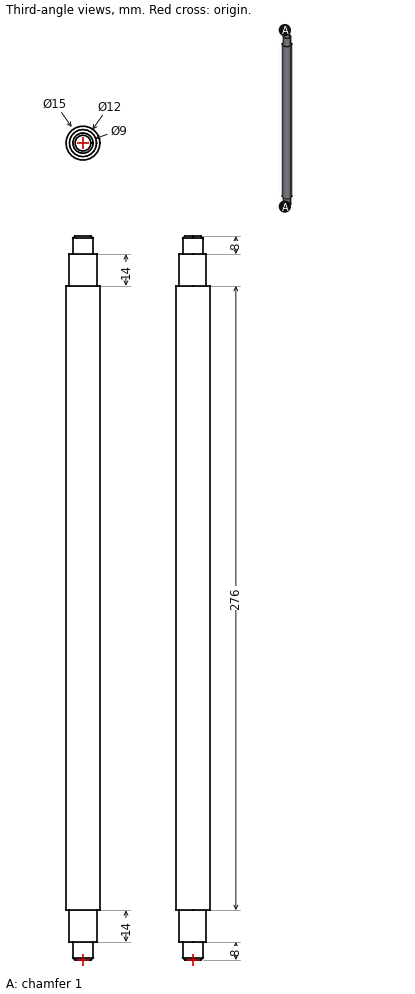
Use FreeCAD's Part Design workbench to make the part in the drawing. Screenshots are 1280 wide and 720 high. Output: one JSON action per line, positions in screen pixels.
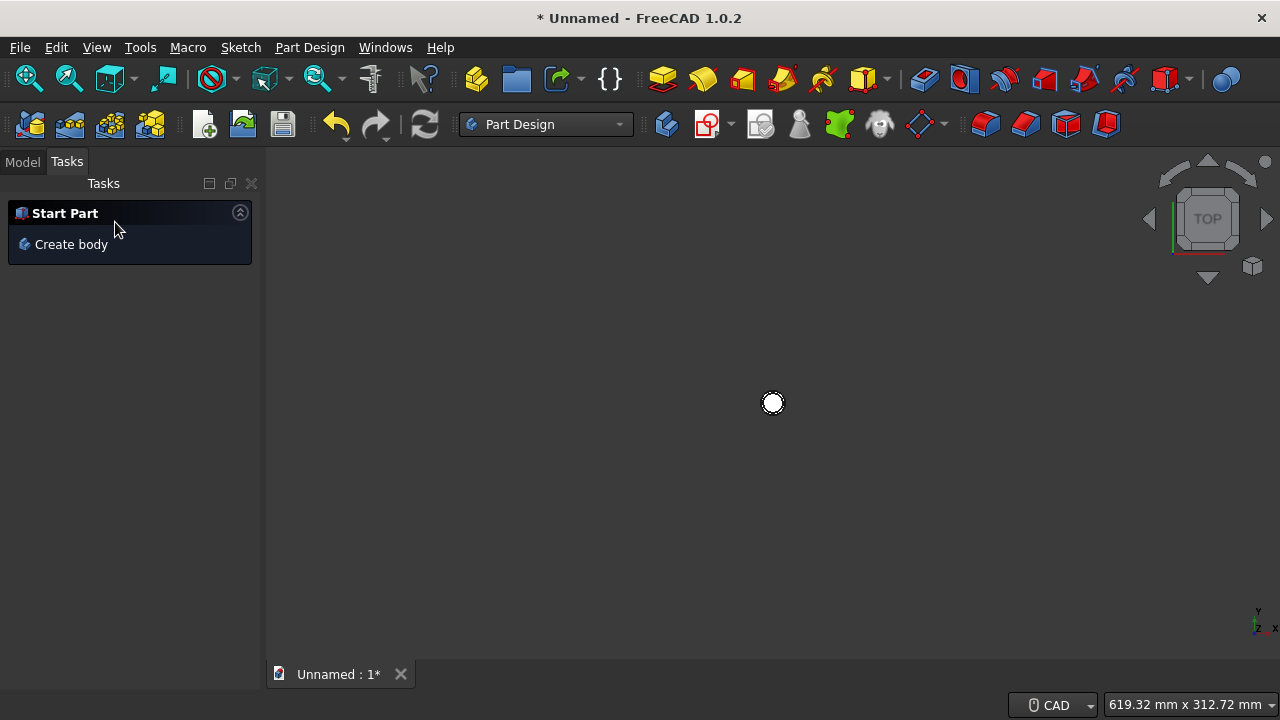
{"action": "left_click", "coordinate": [773, 402]}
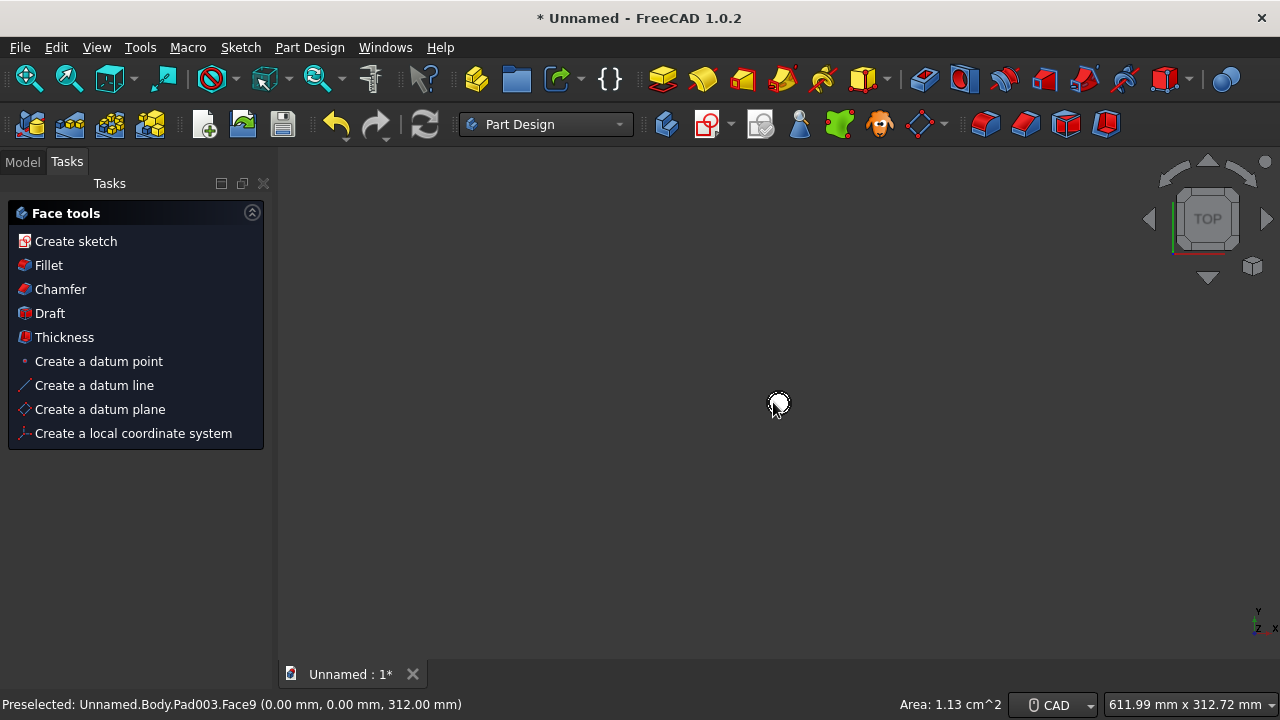
{"action": "left_click", "coordinate": [708, 124]}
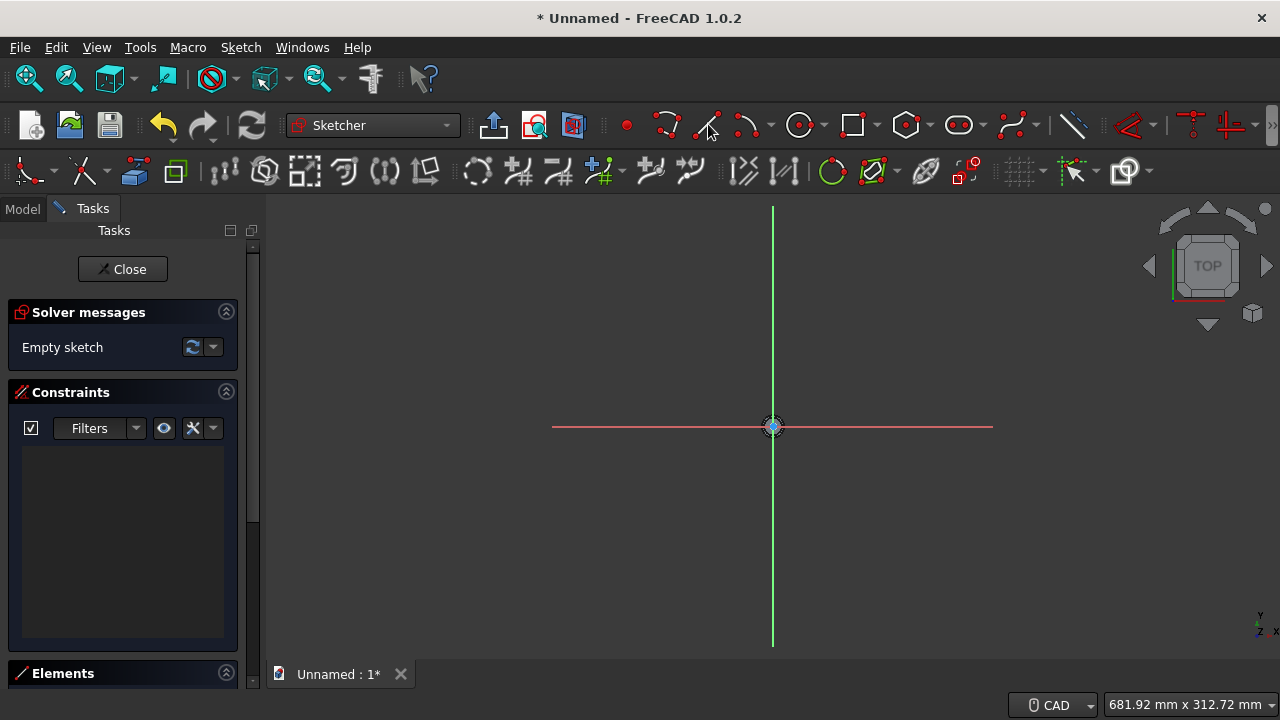
{"action": "scroll", "coordinate": [777, 426], "scroll_direction": "up", "scroll_amount": 15}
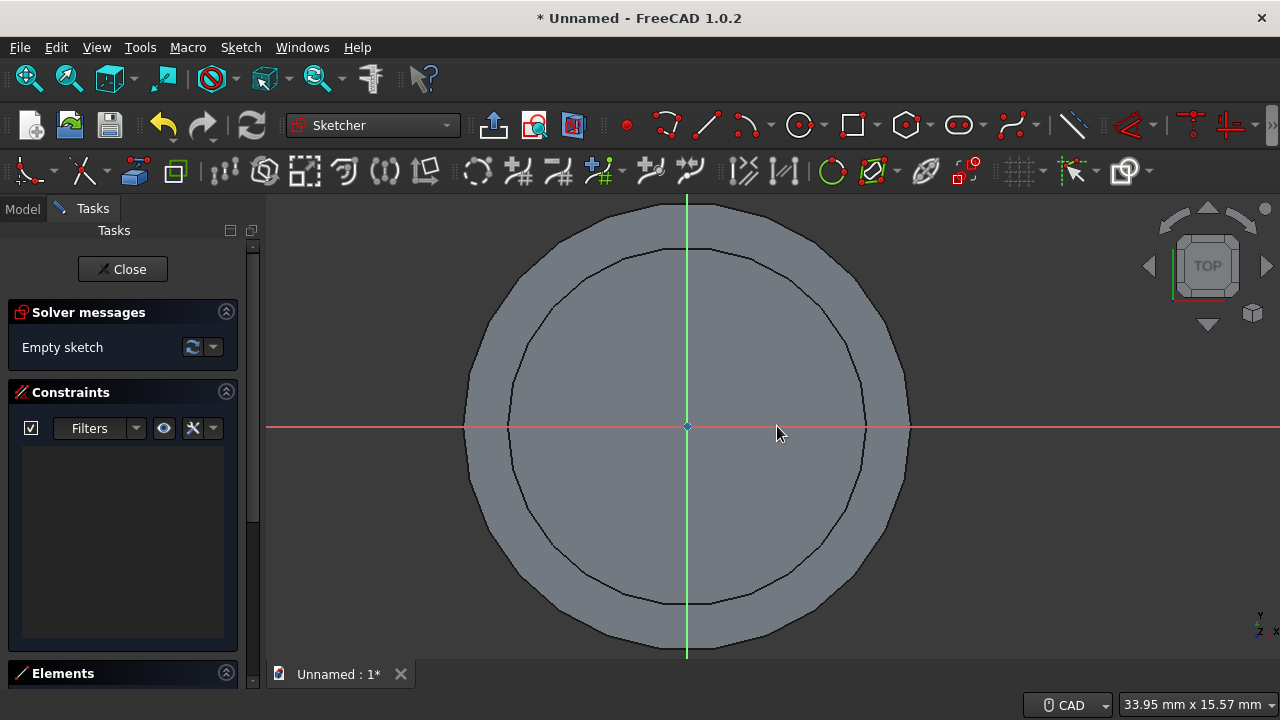
{"action": "left_click", "coordinate": [800, 126]}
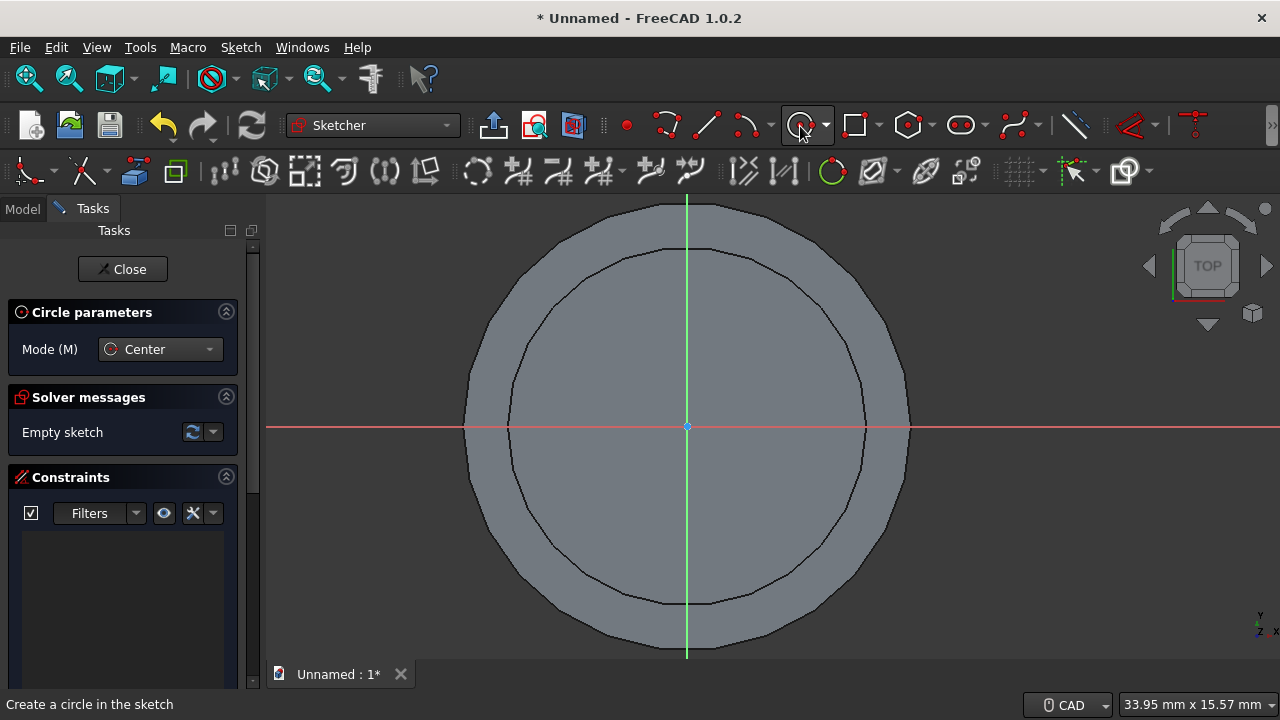
{"action": "left_click", "coordinate": [687, 426]}
{"action": "left_click", "coordinate": [782, 331]}
{"action": "key", "text": "Escape"}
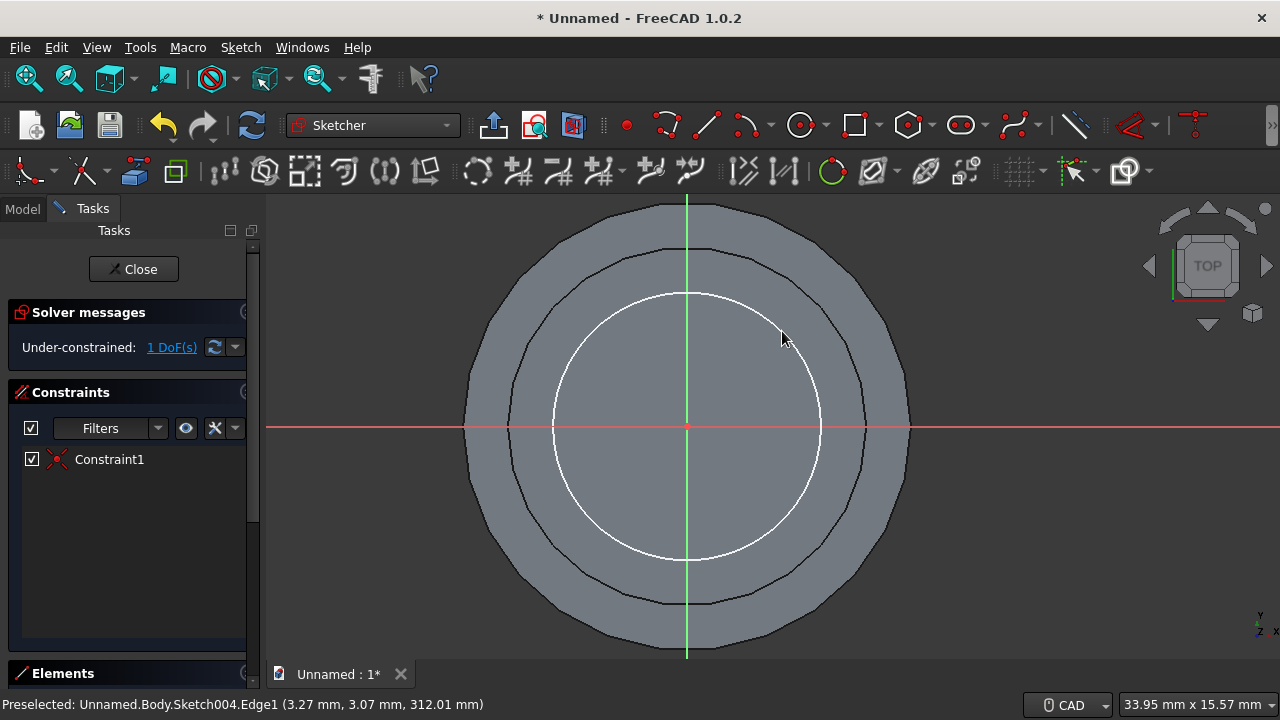
{"action": "left_click", "coordinate": [1130, 126]}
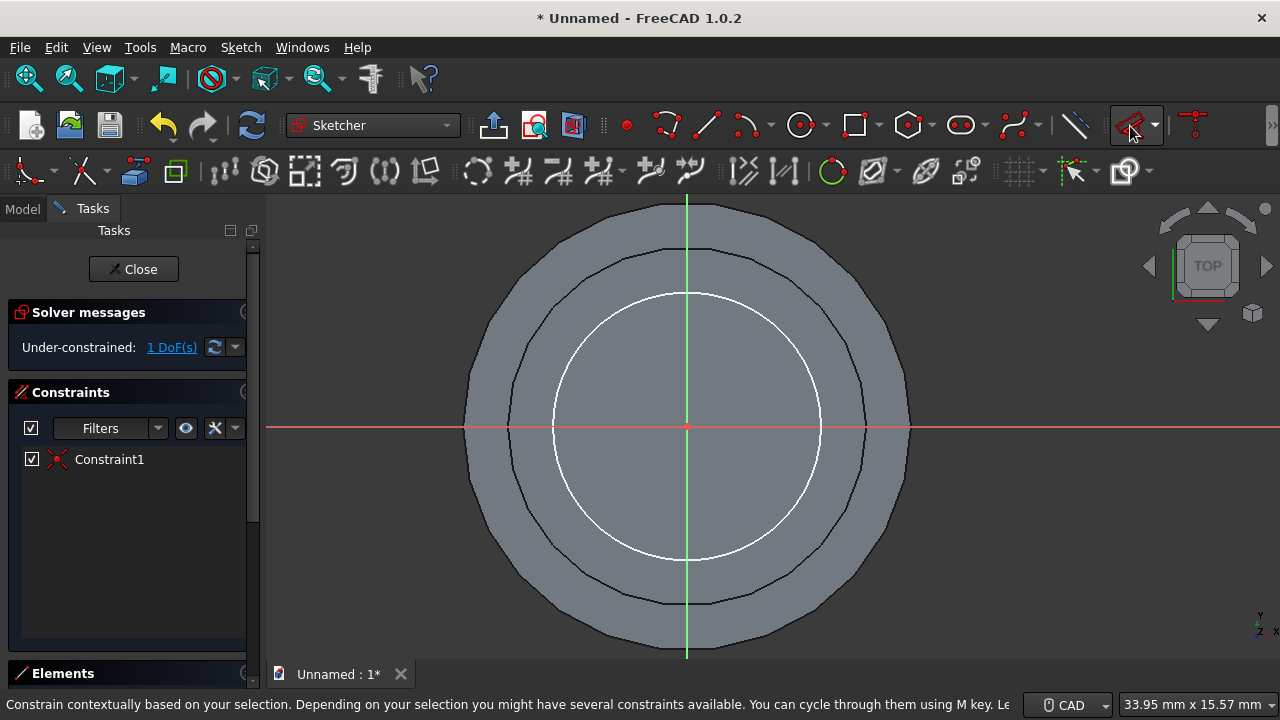
{"action": "left_click", "coordinate": [781, 331]}
{"action": "left_click", "coordinate": [803, 308]}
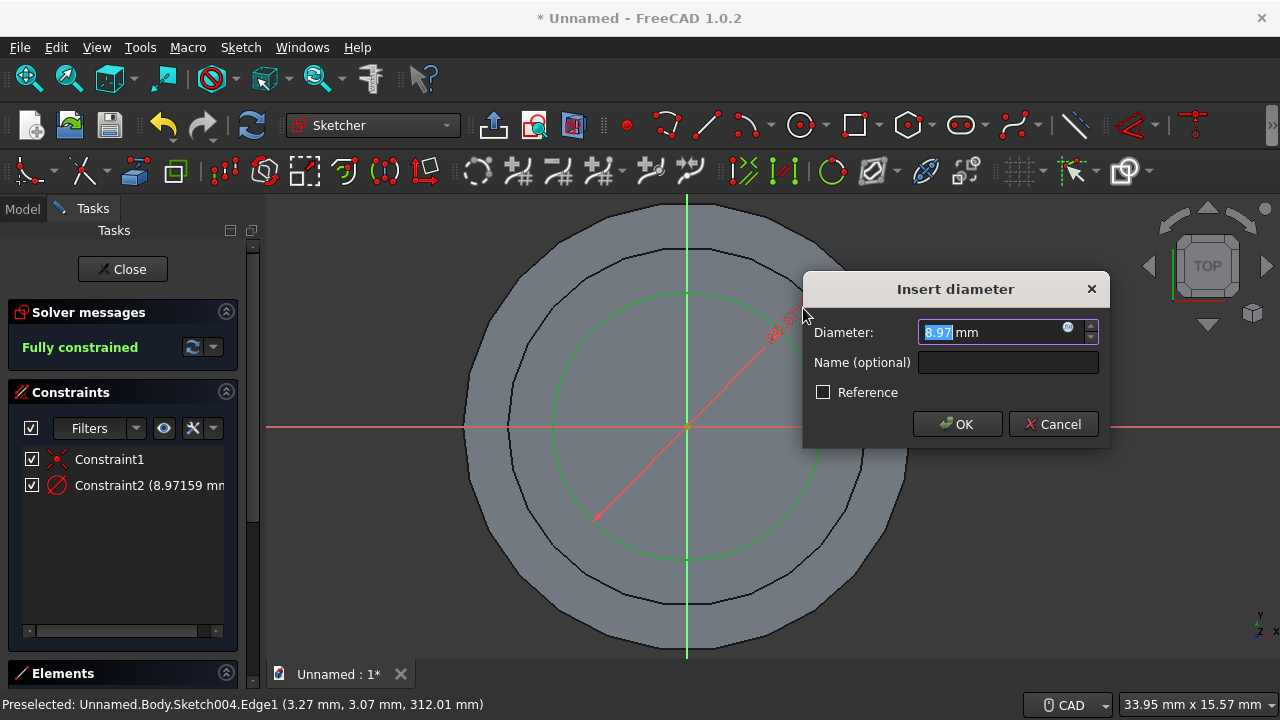
{"action": "type", "text": "9"}
{"action": "key", "text": "Return"}
{"action": "key", "text": "Escape"}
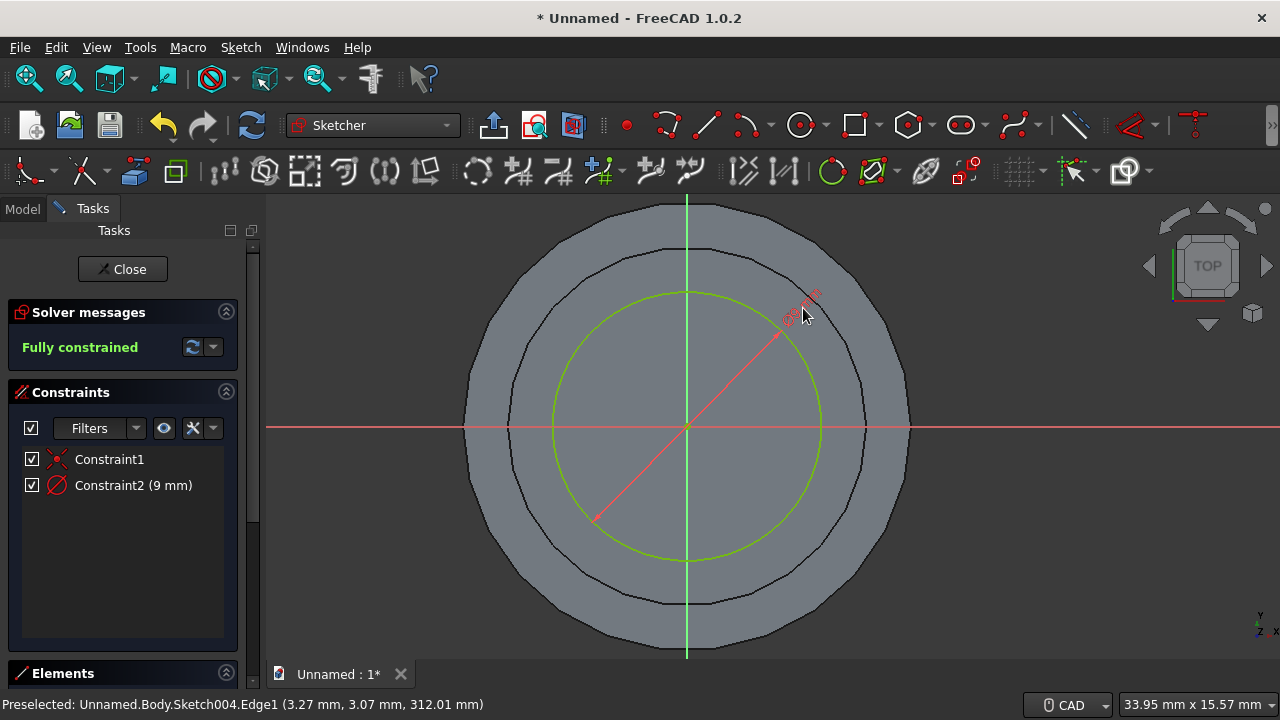
{"action": "left_click", "coordinate": [123, 269]}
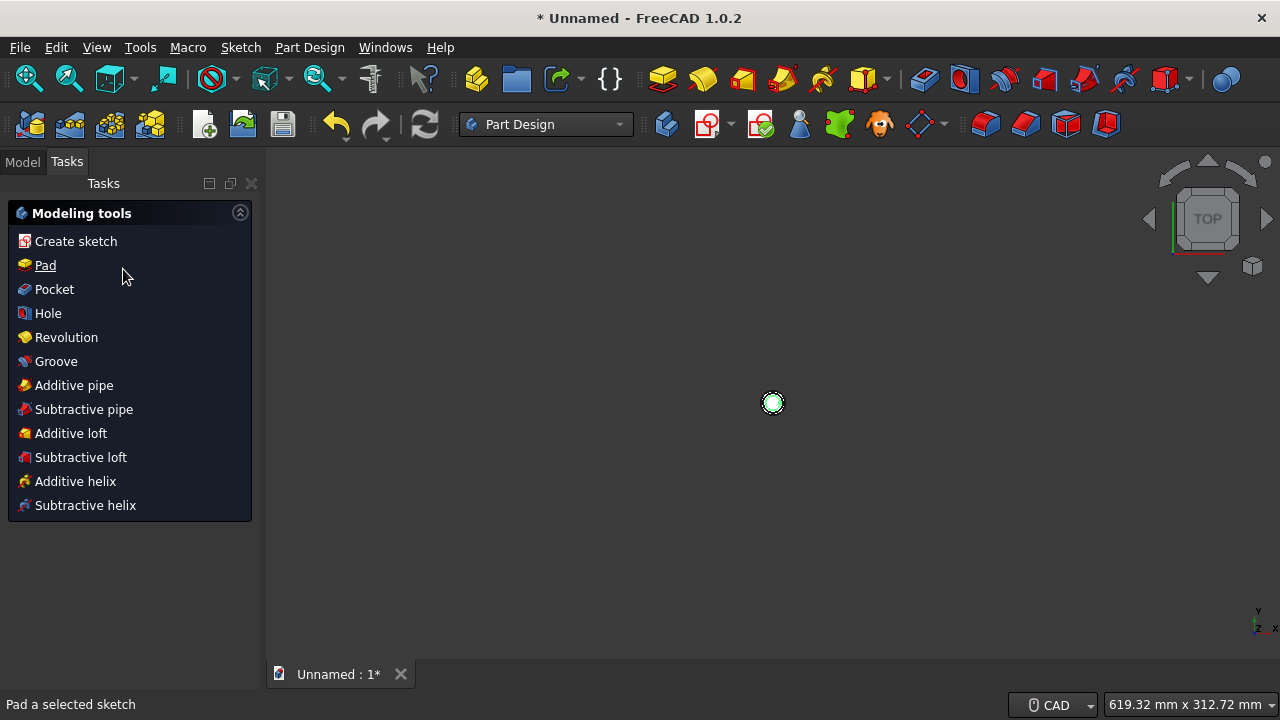
{"action": "left_click", "coordinate": [664, 80]}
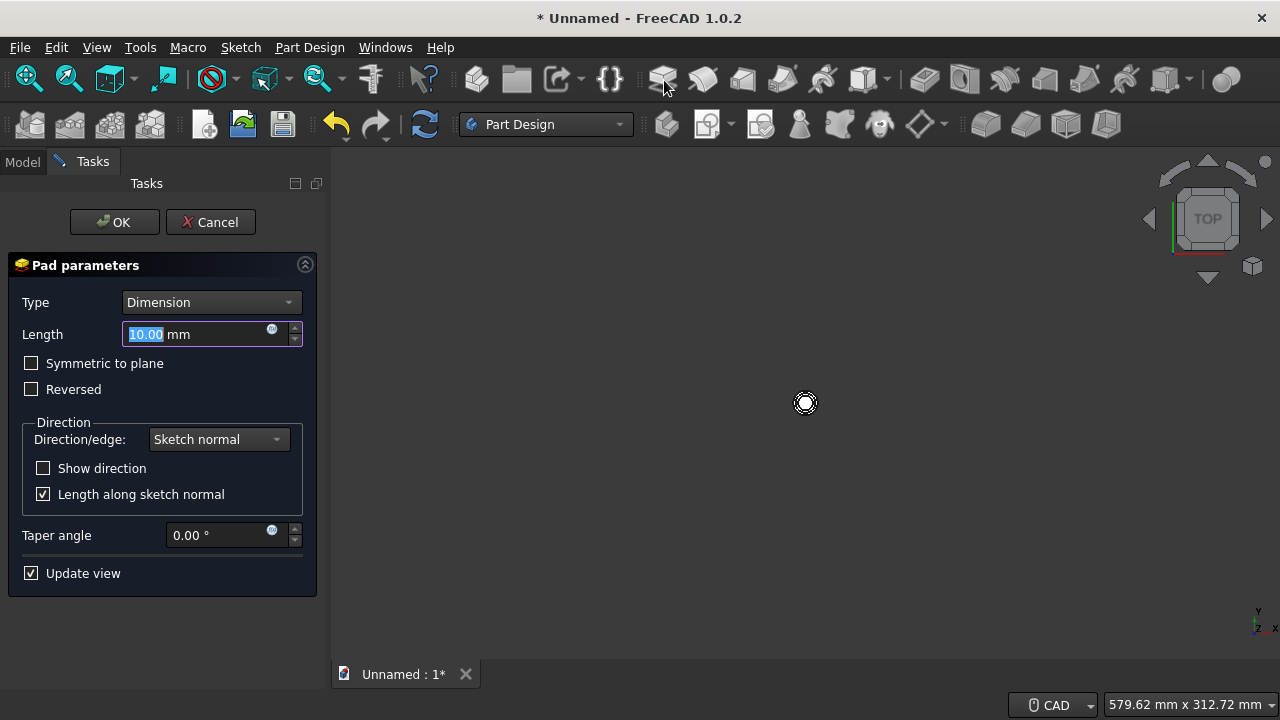
{"action": "type", "text": "8"}
{"action": "key", "text": "Tab"}